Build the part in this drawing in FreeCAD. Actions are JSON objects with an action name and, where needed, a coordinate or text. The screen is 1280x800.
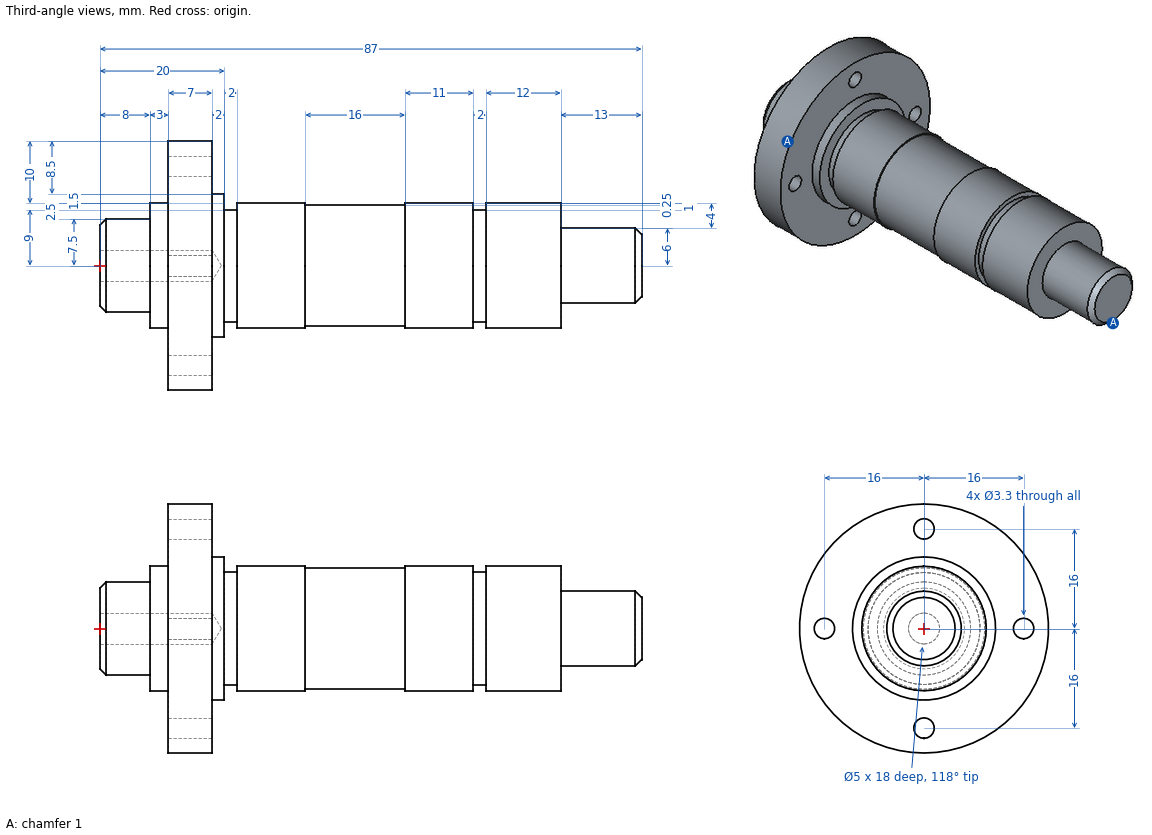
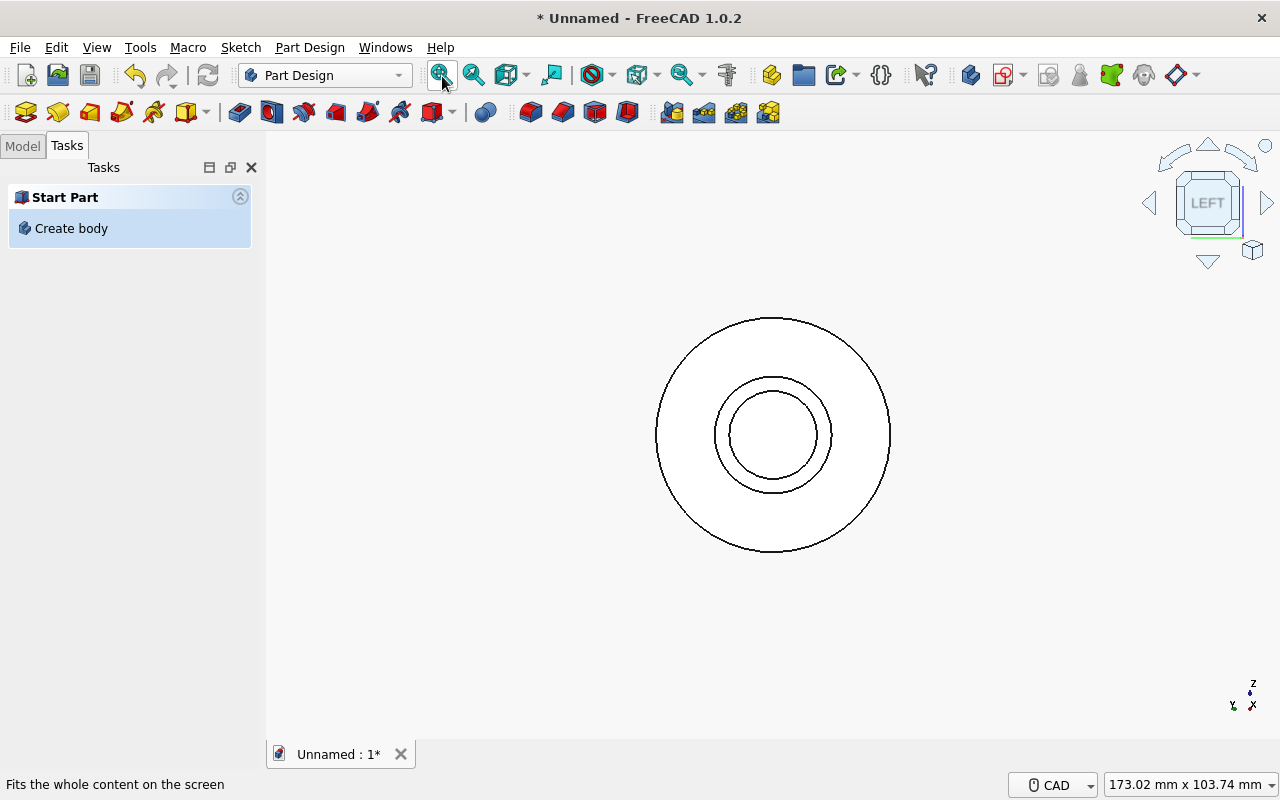
{"action": "left_click", "coordinate": [442, 76]}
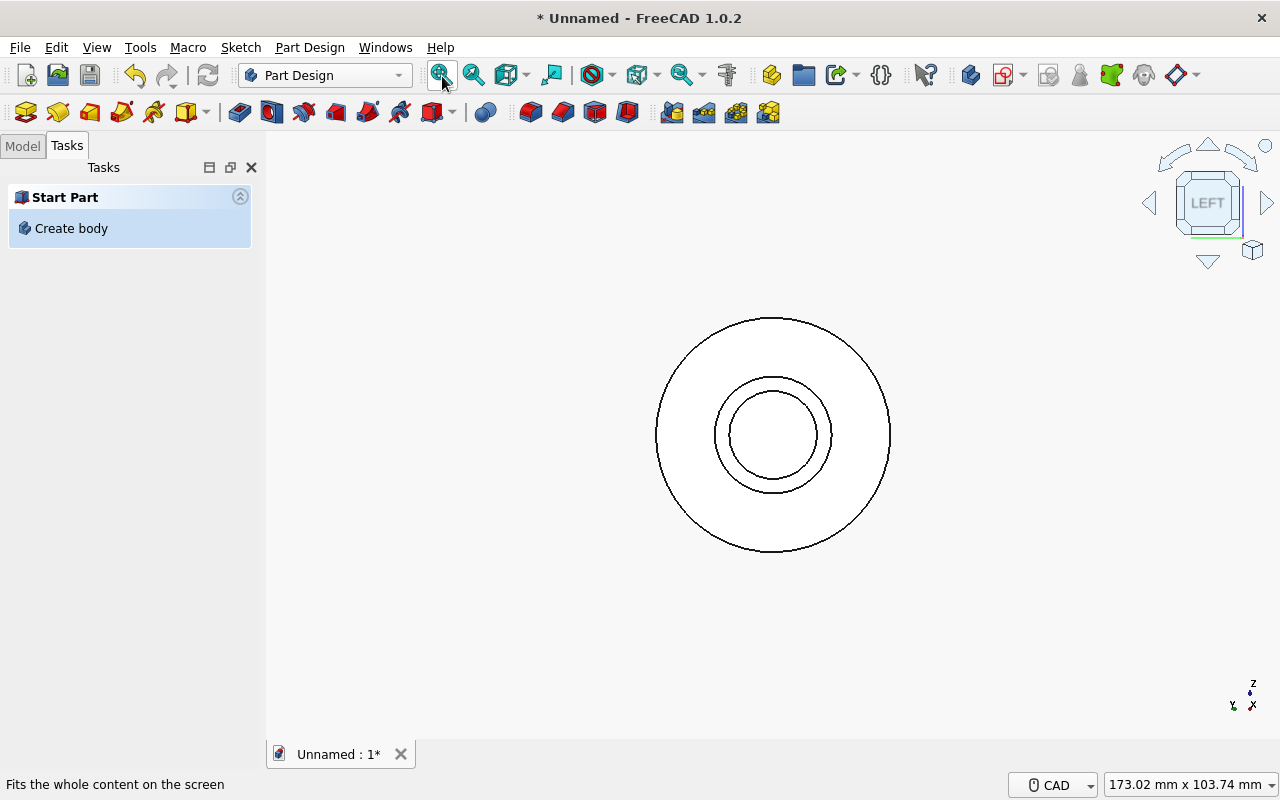
{"action": "left_click", "coordinate": [773, 434]}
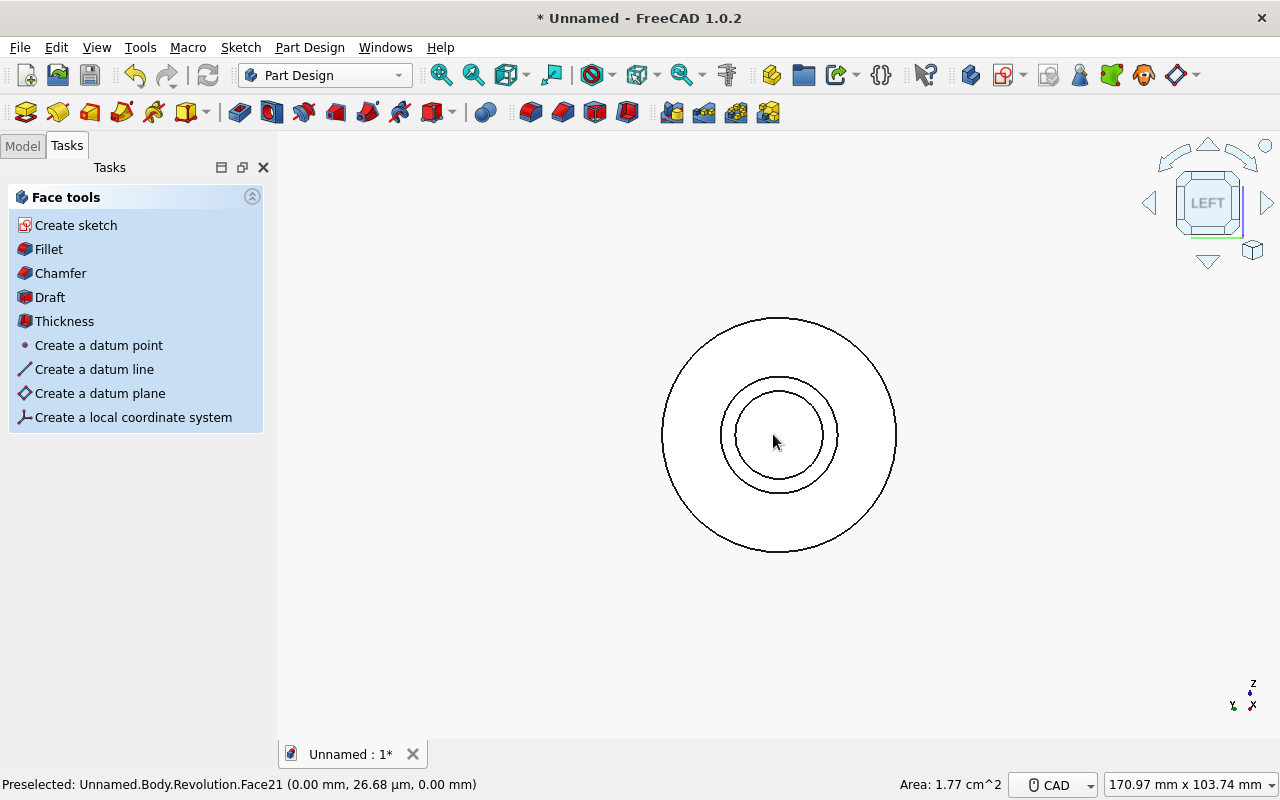
{"action": "left_click", "coordinate": [1004, 76]}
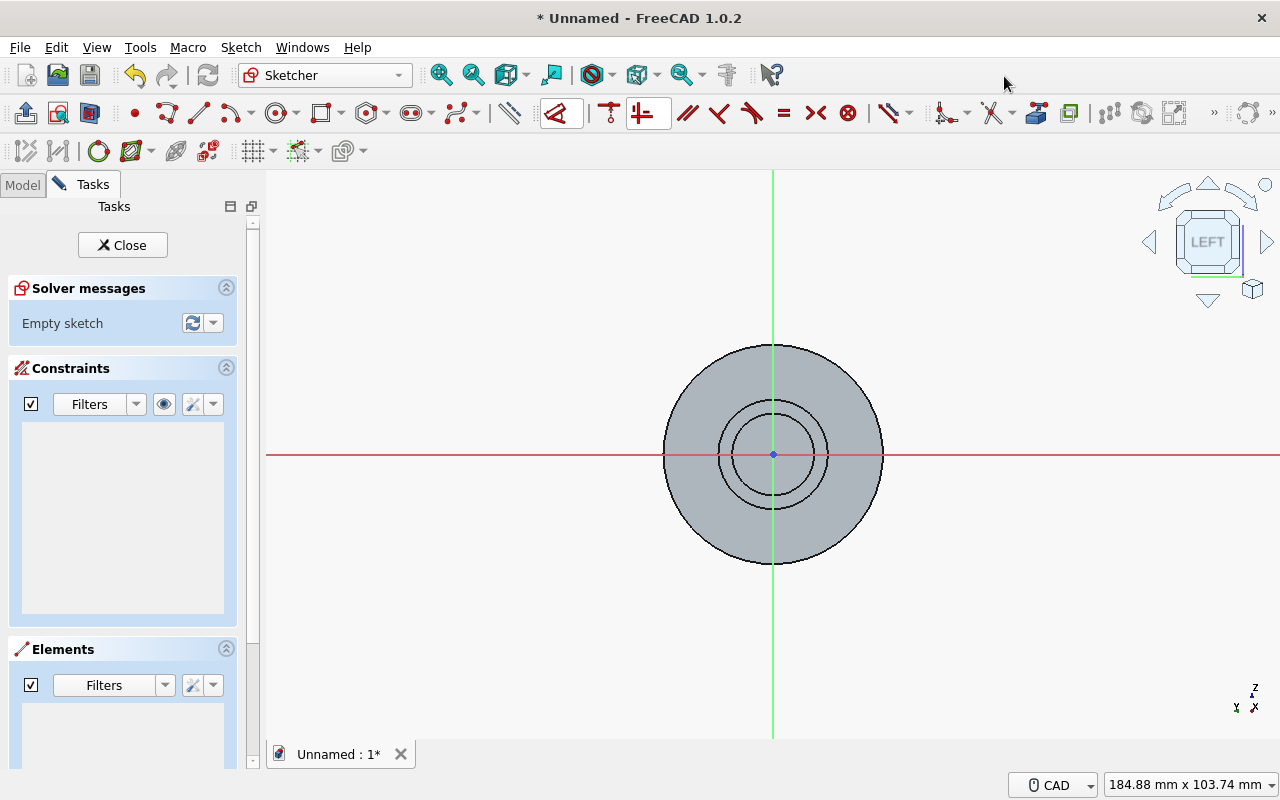
{"action": "scroll", "coordinate": [779, 454], "scroll_direction": "up", "scroll_amount": 13}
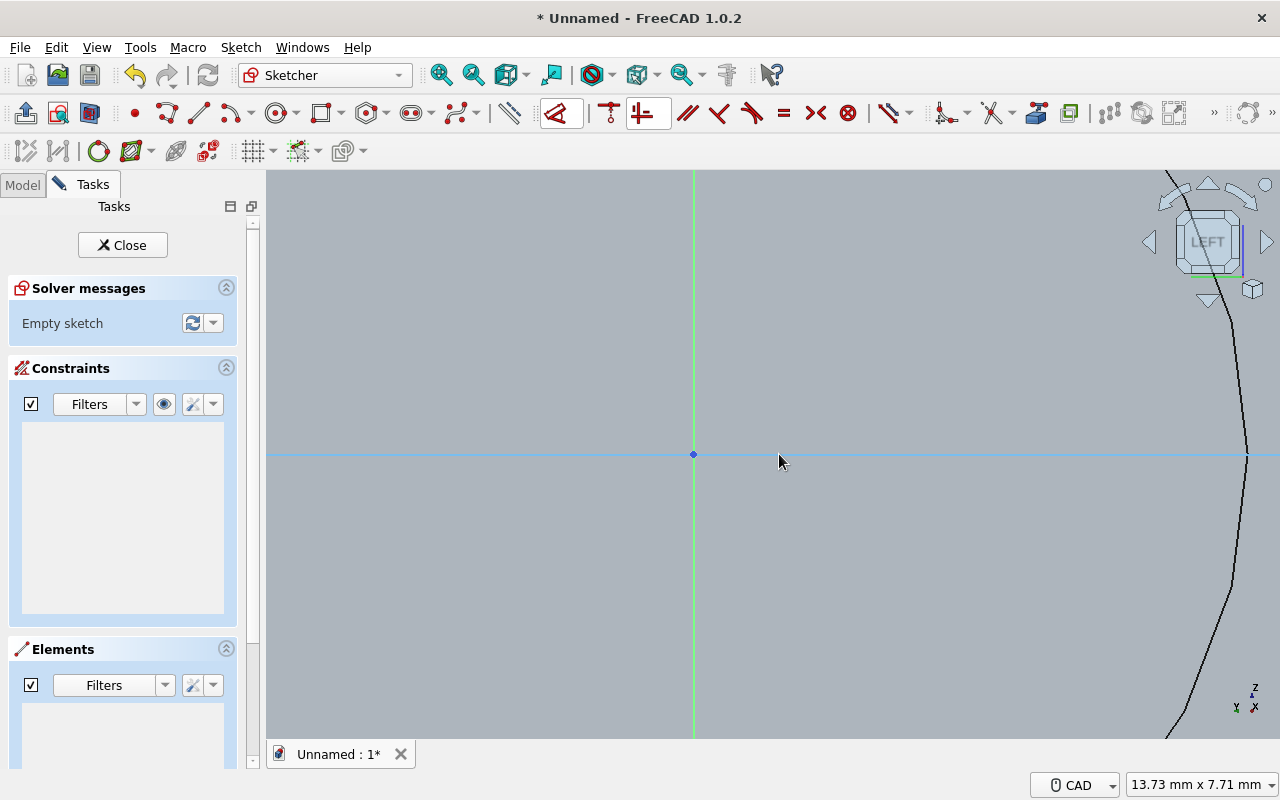
{"action": "left_click", "coordinate": [276, 114]}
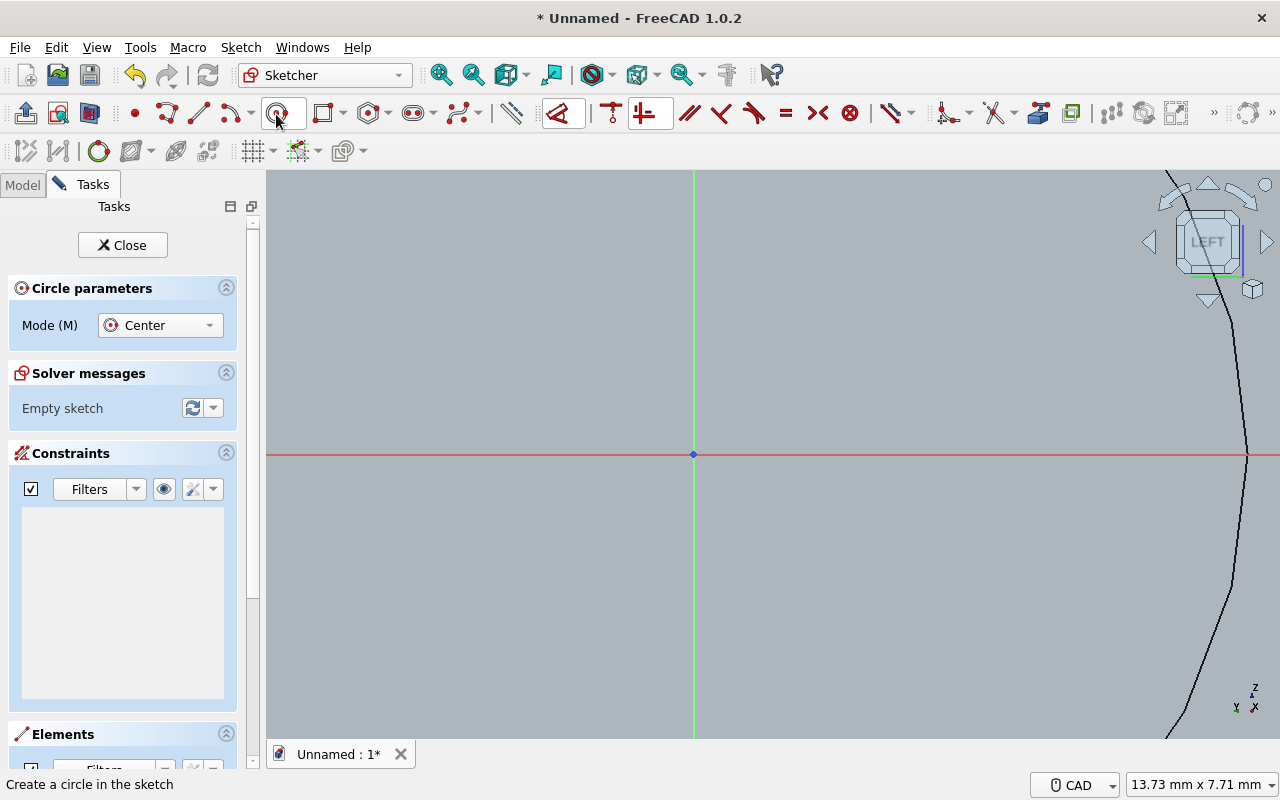
{"action": "left_click", "coordinate": [694, 454]}
{"action": "mouse_move", "coordinate": [824, 324]}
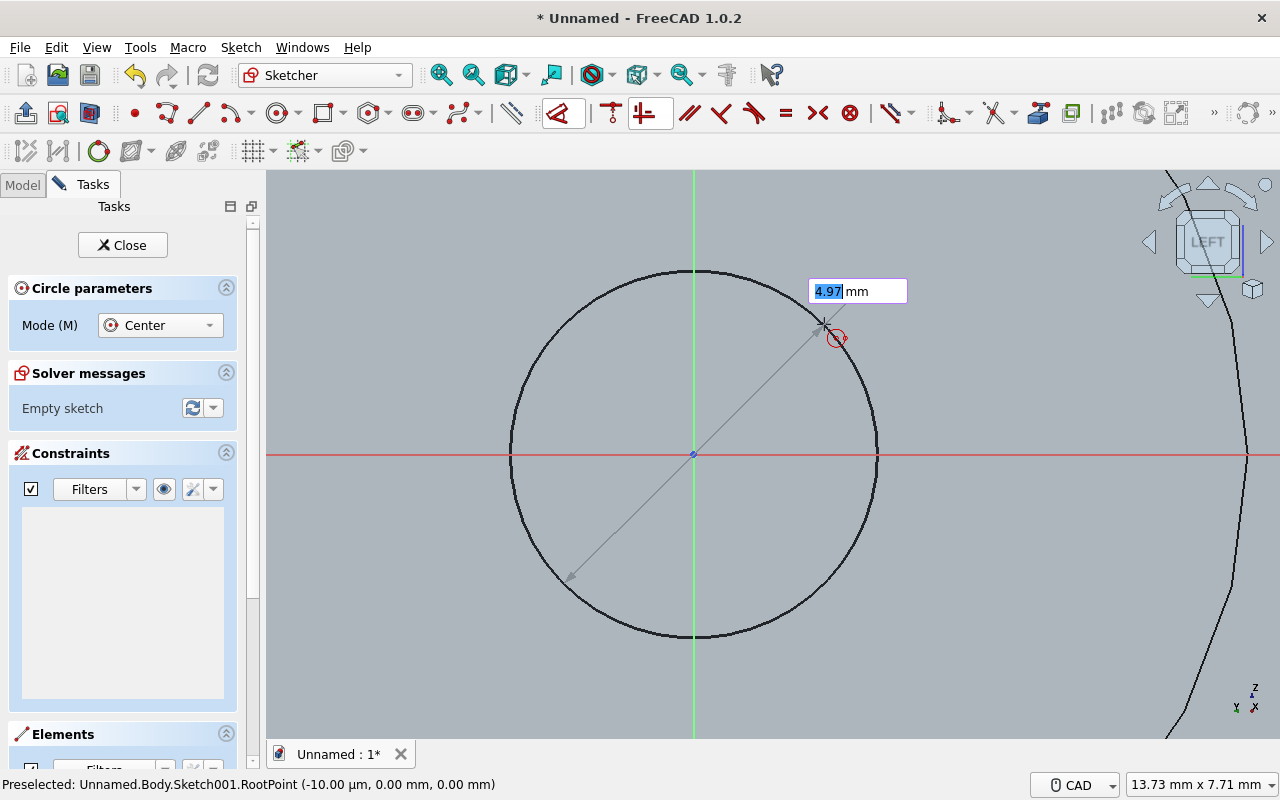
{"action": "type", "text": "5"}
{"action": "key", "text": "Return"}
{"action": "key", "text": "Escape"}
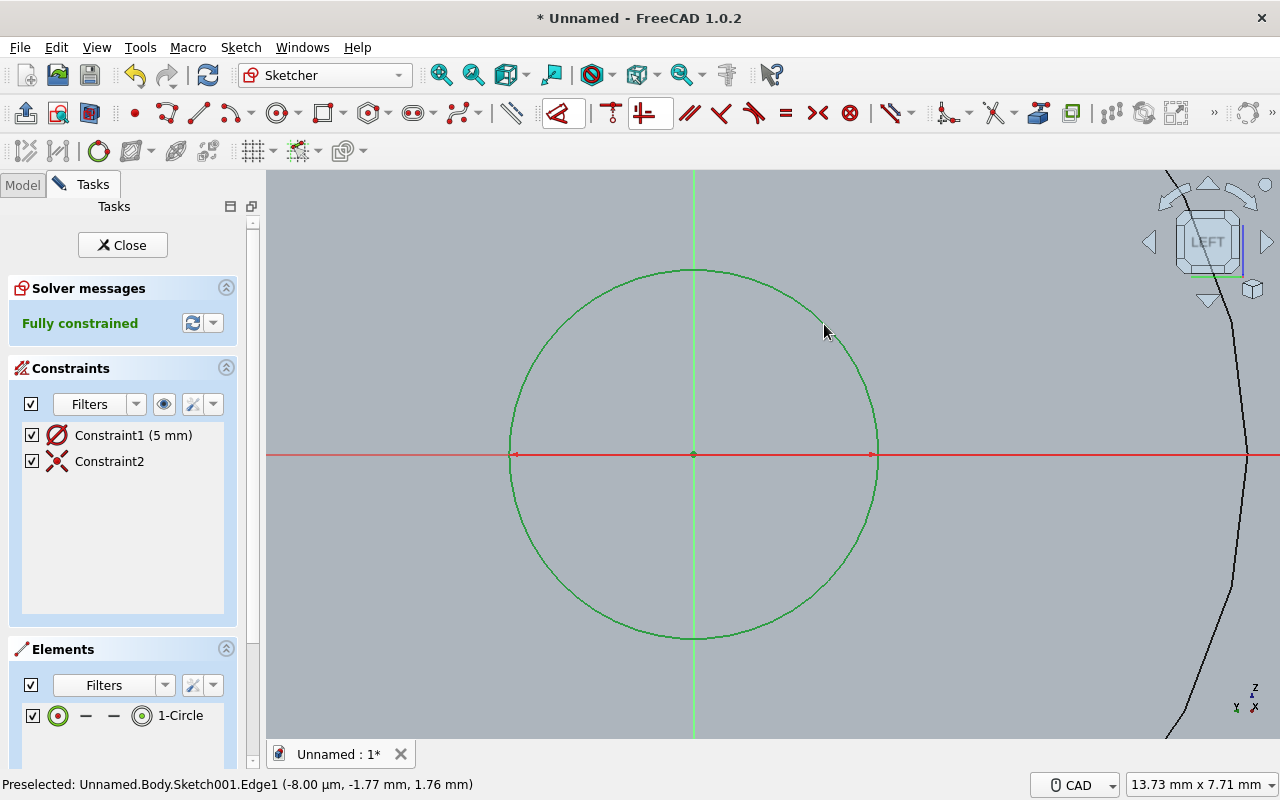
{"action": "left_click", "coordinate": [123, 245]}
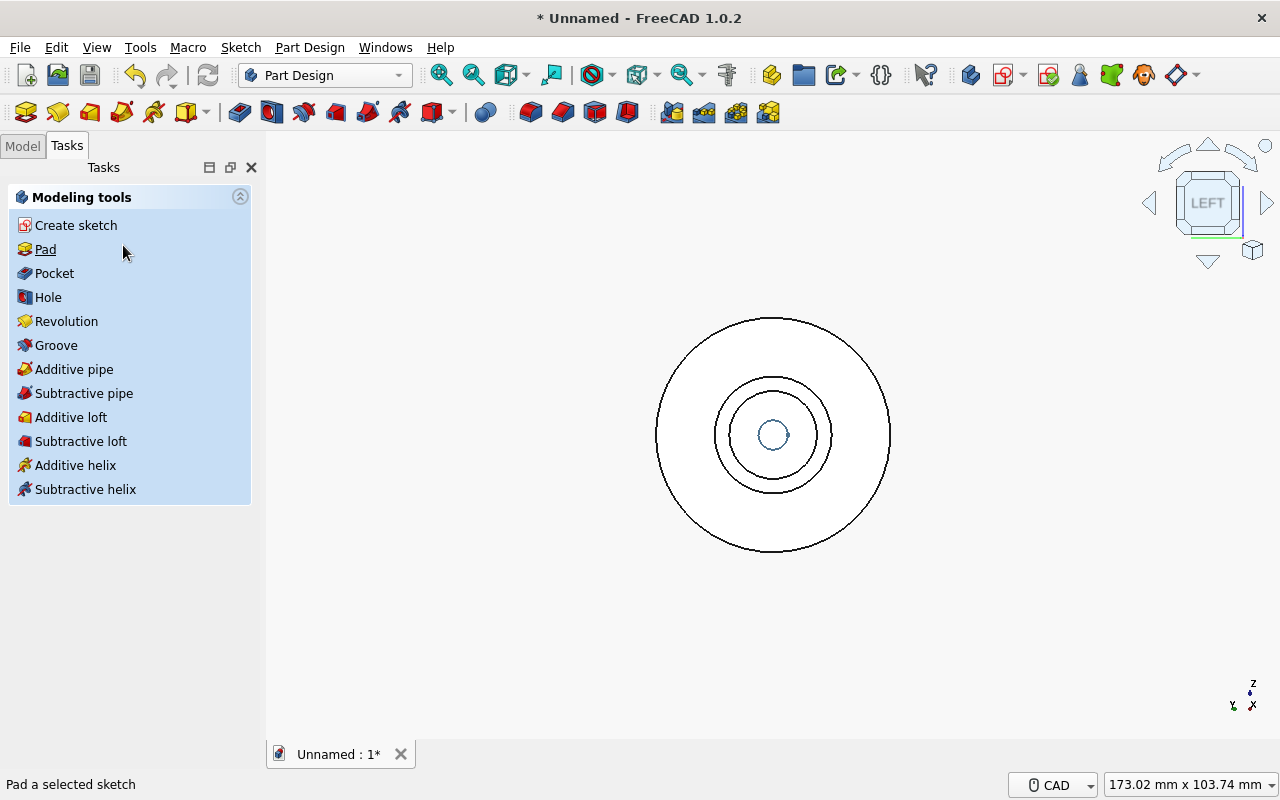
{"action": "left_click", "coordinate": [272, 112]}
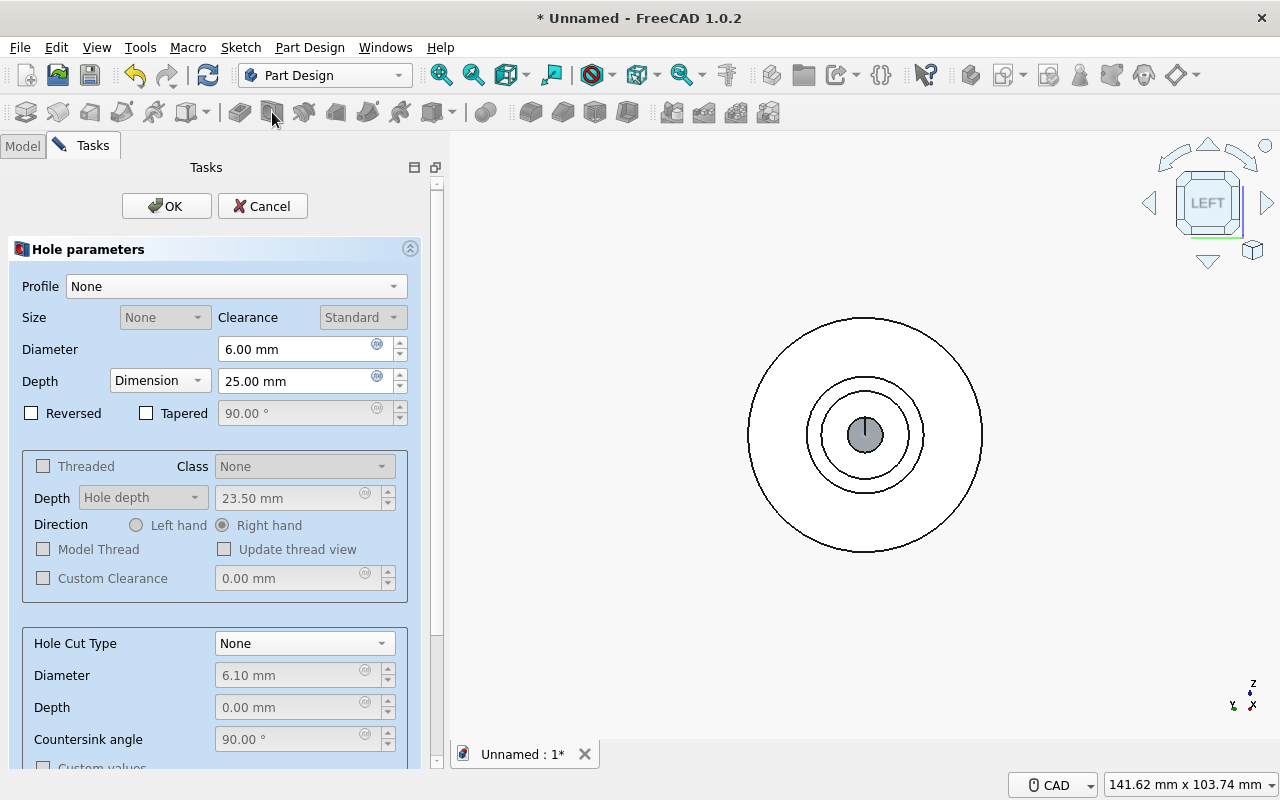
{"action": "triple_click", "coordinate": [305, 349]}